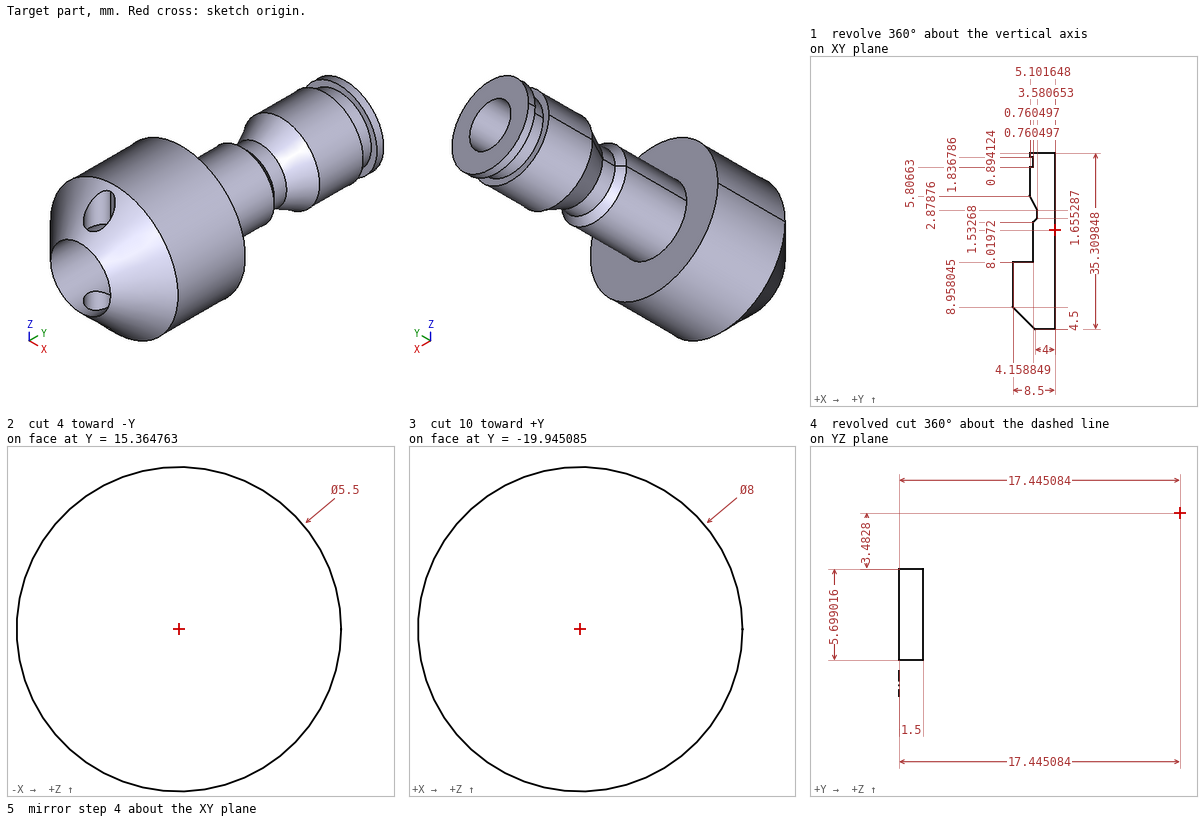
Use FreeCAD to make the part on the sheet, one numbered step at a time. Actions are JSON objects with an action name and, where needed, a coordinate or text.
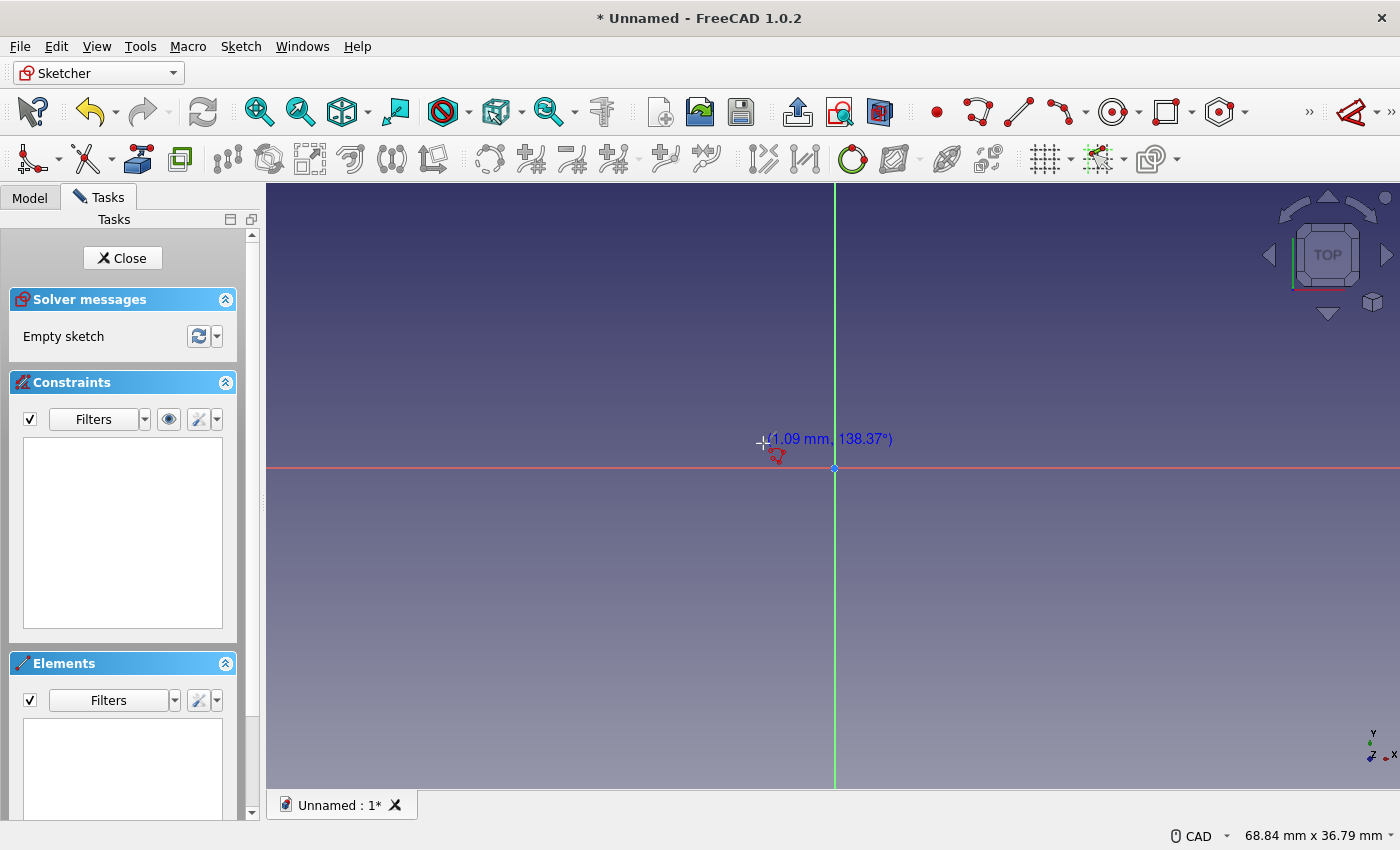
{"action": "left_click", "coordinate": [763, 443]}
{"action": "left_click", "coordinate": [763, 575]}
{"action": "left_click", "coordinate": [695, 575]}
{"action": "left_click", "coordinate": [695, 723]}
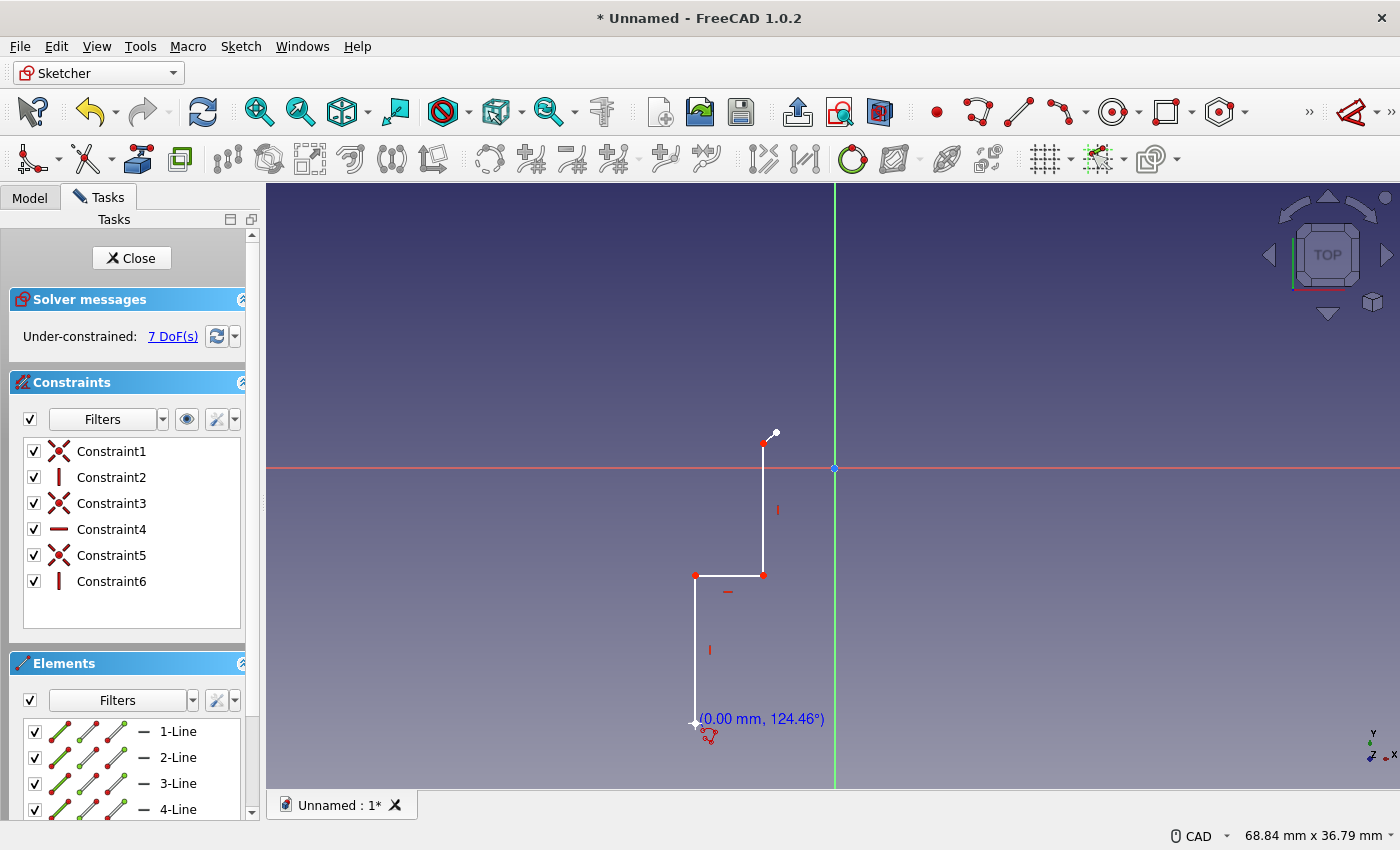
{"action": "scroll", "coordinate": [764, 445], "scroll_direction": "down", "scroll_amount": 2}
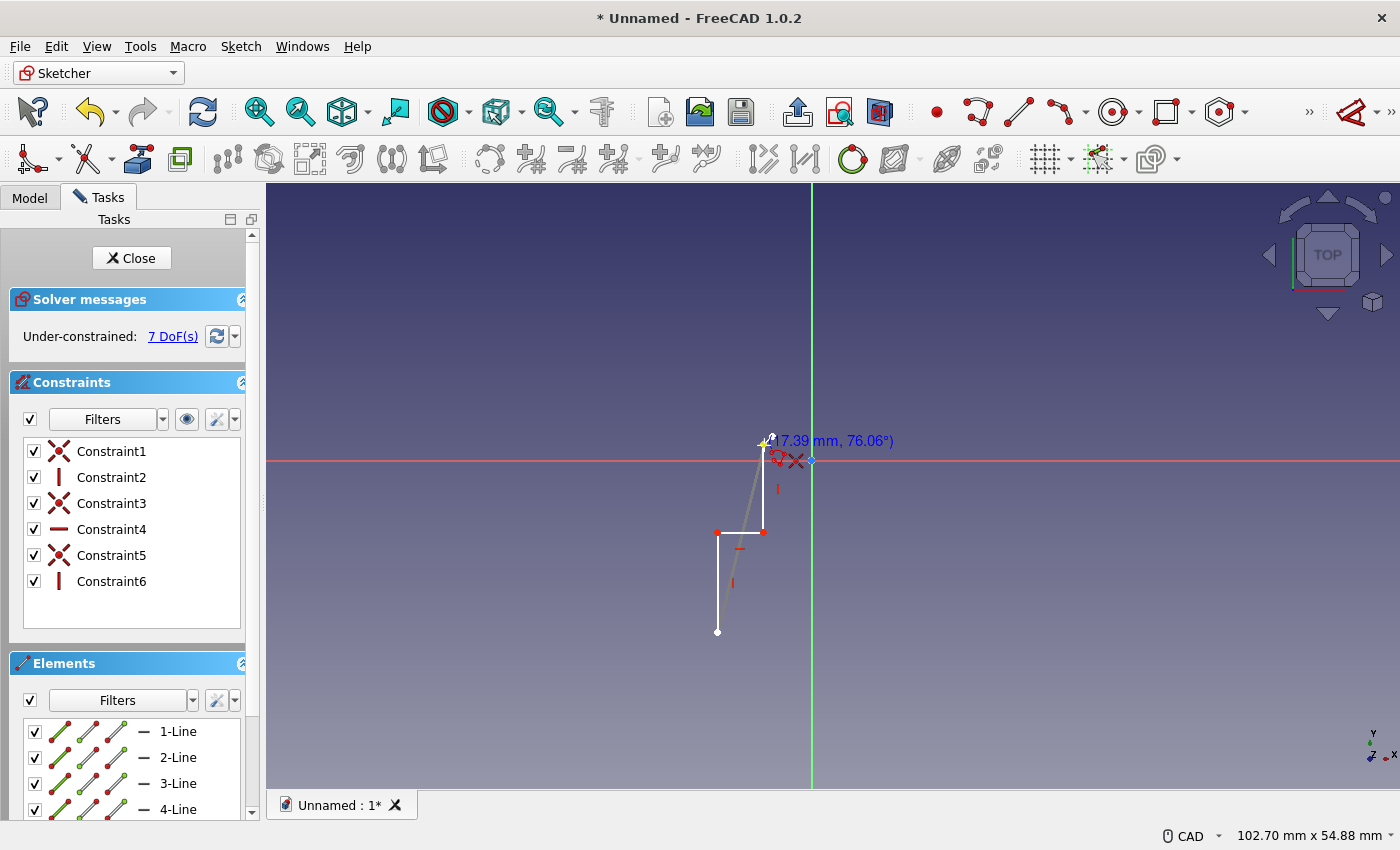
{"action": "left_click", "coordinate": [767, 681]}
{"action": "left_click", "coordinate": [812, 681]}
{"action": "left_click", "coordinate": [803, 291]}
{"action": "left_click", "coordinate": [755, 291]}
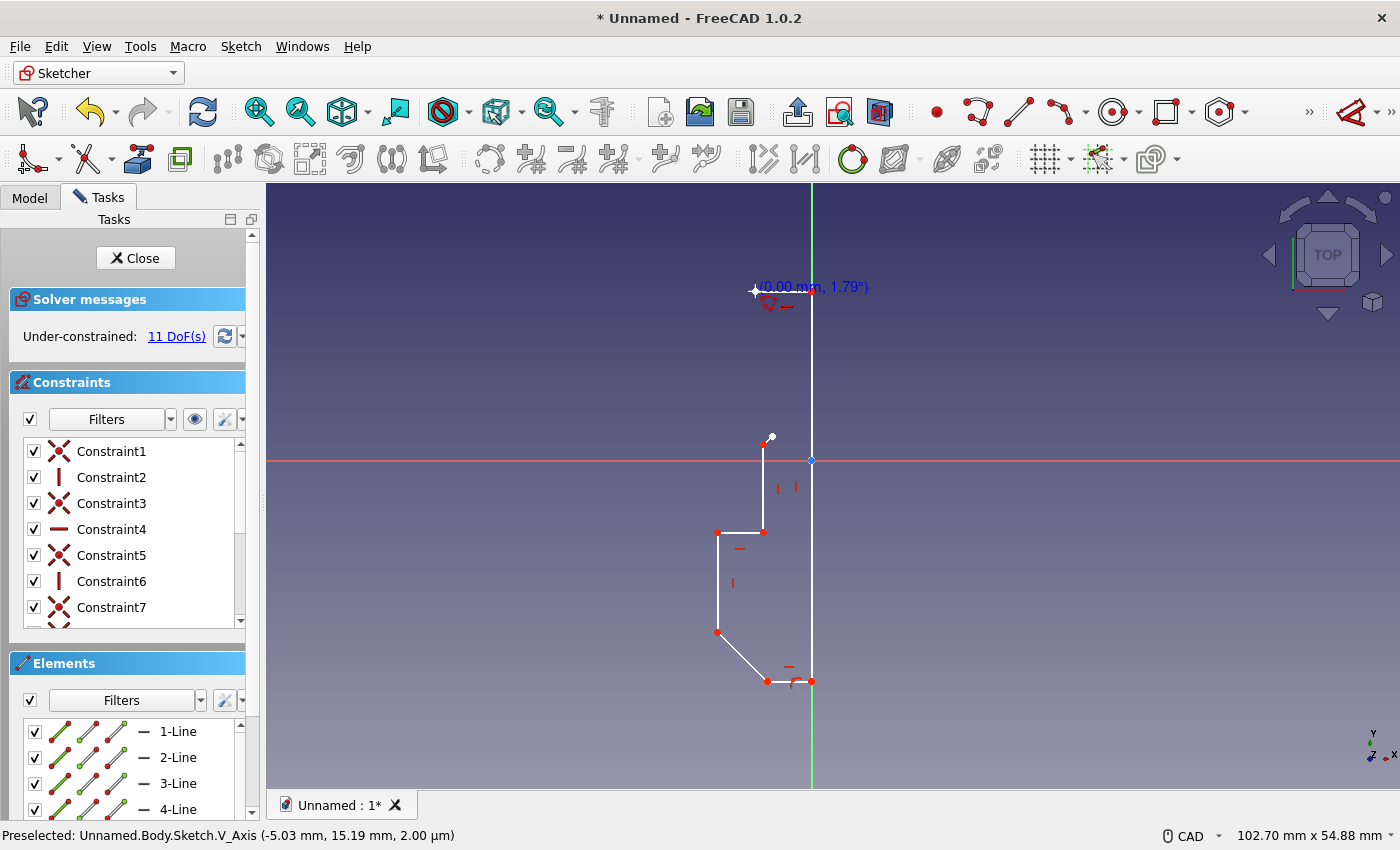
{"action": "scroll", "coordinate": [755, 301], "scroll_direction": "up", "scroll_amount": 3}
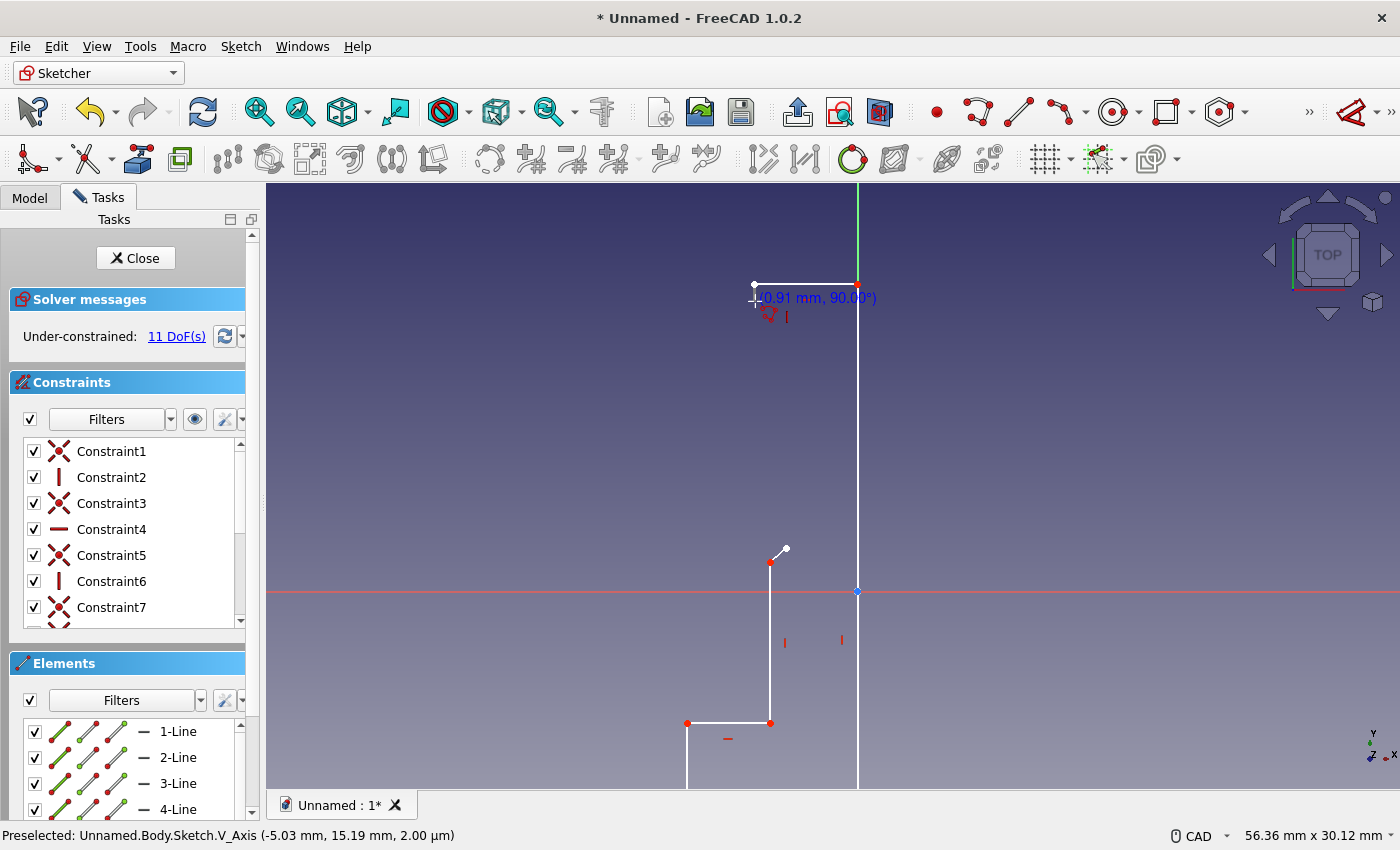
{"action": "left_click", "coordinate": [755, 301]}
{"action": "left_click", "coordinate": [770, 301]}
{"action": "left_click", "coordinate": [770, 338]}
{"action": "left_click", "coordinate": [755, 338]}
{"action": "left_click", "coordinate": [755, 455]}
{"action": "left_click", "coordinate": [786, 512]}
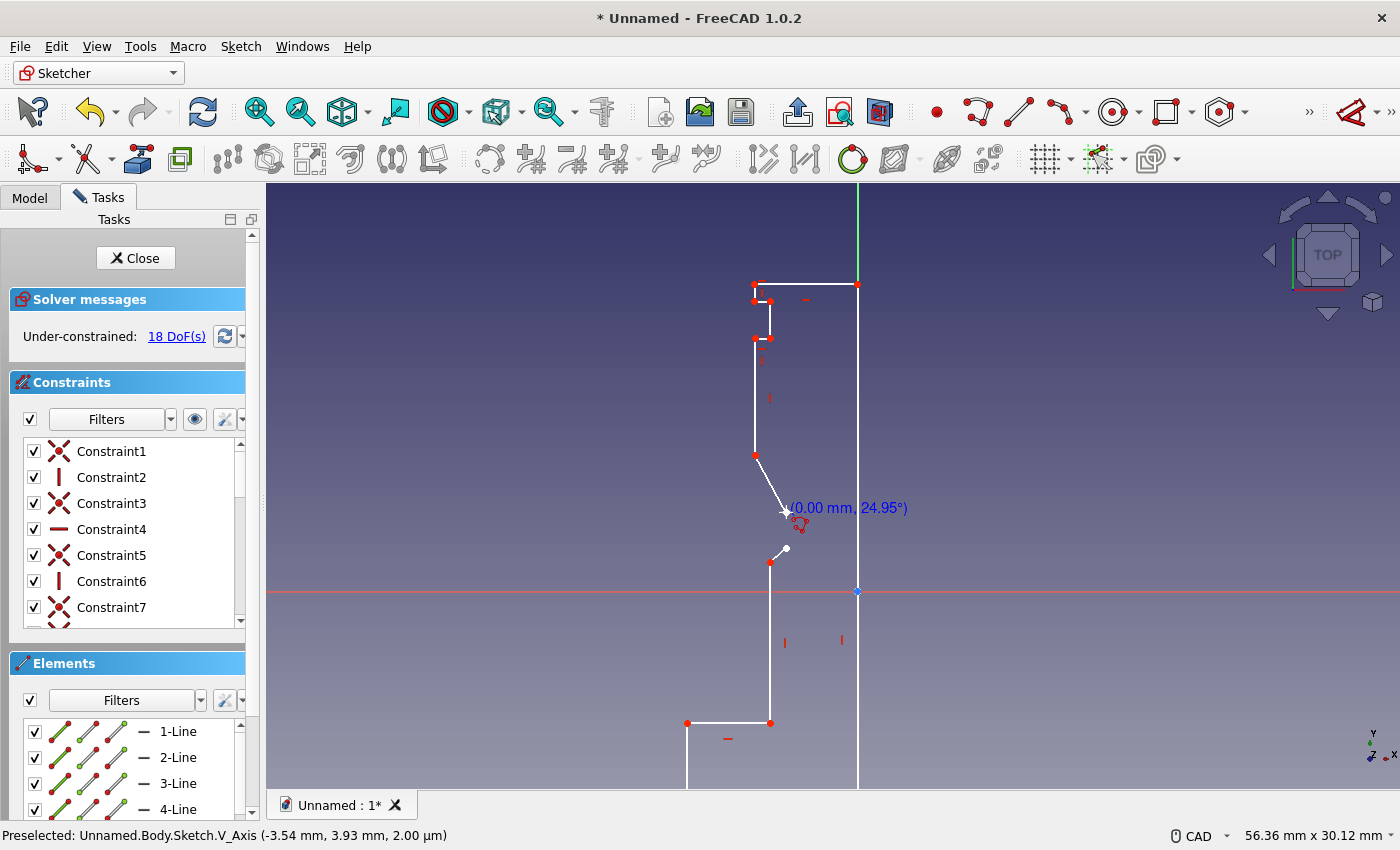
{"action": "scroll", "coordinate": [786, 546], "scroll_direction": "up", "scroll_amount": 2}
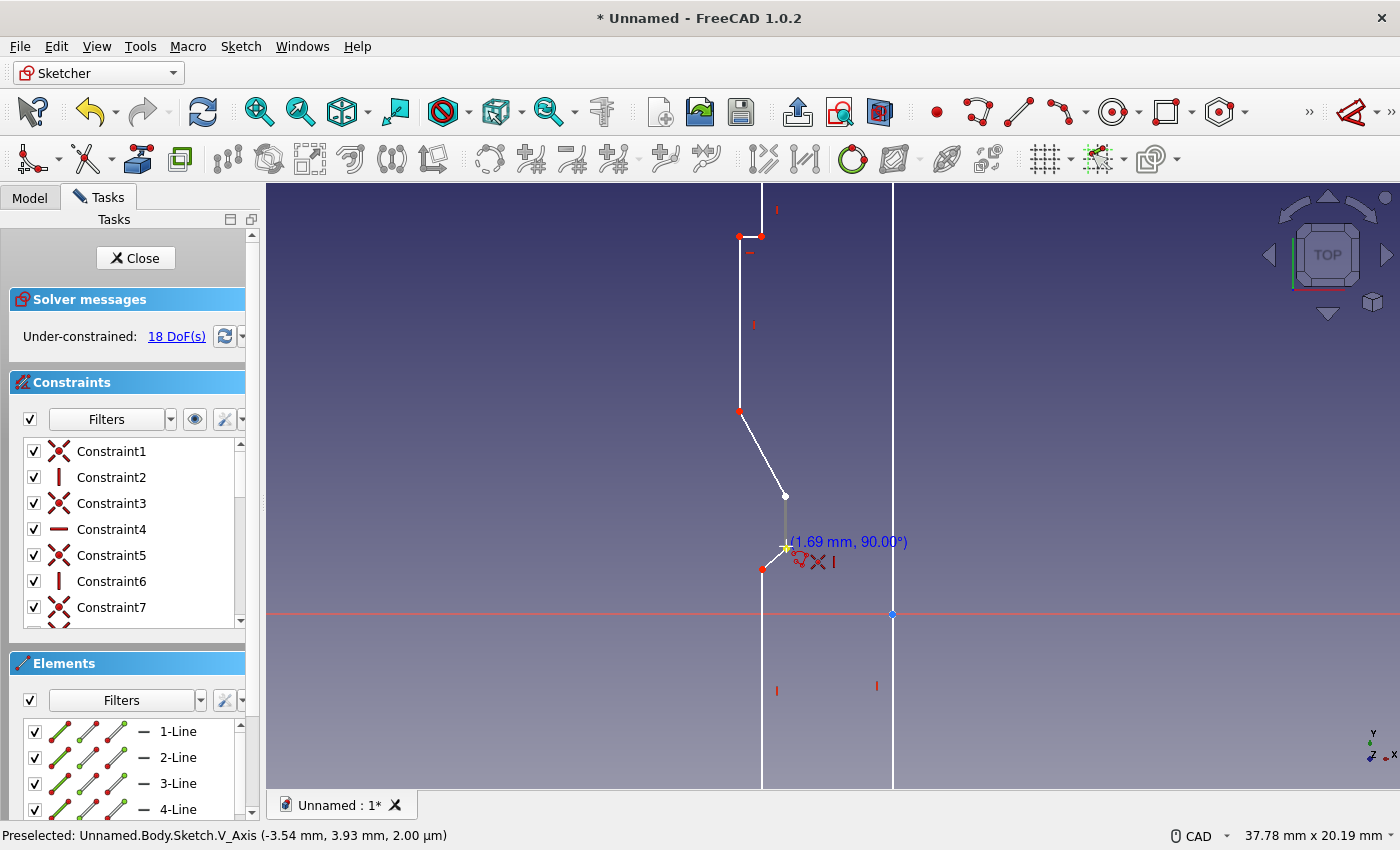
{"action": "left_click", "coordinate": [786, 549]}
{"action": "key", "text": "Escape"}
{"action": "key", "text": "Escape"}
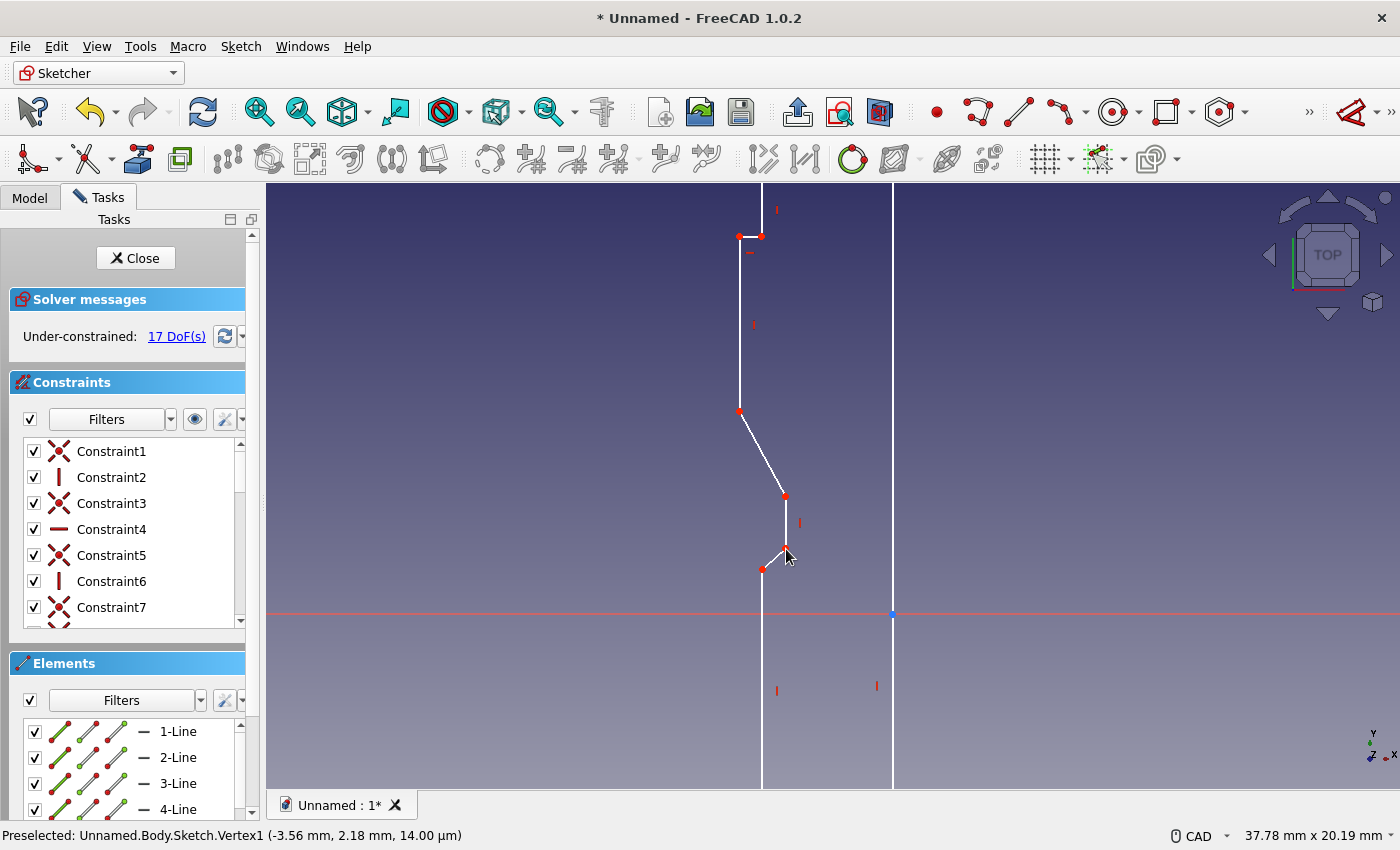
{"action": "left_click", "coordinate": [1350, 112]}